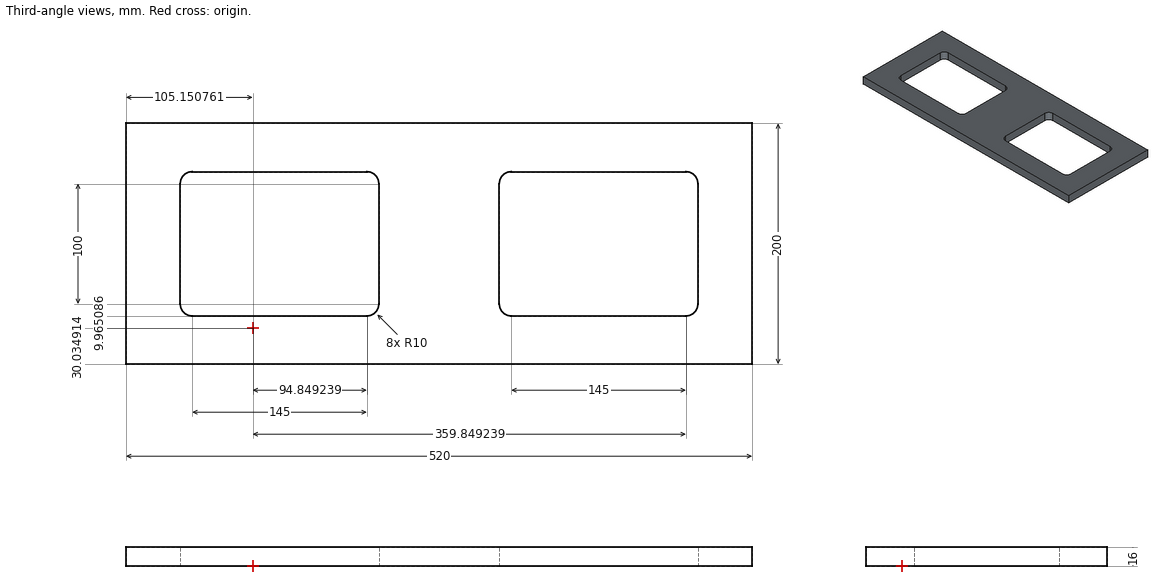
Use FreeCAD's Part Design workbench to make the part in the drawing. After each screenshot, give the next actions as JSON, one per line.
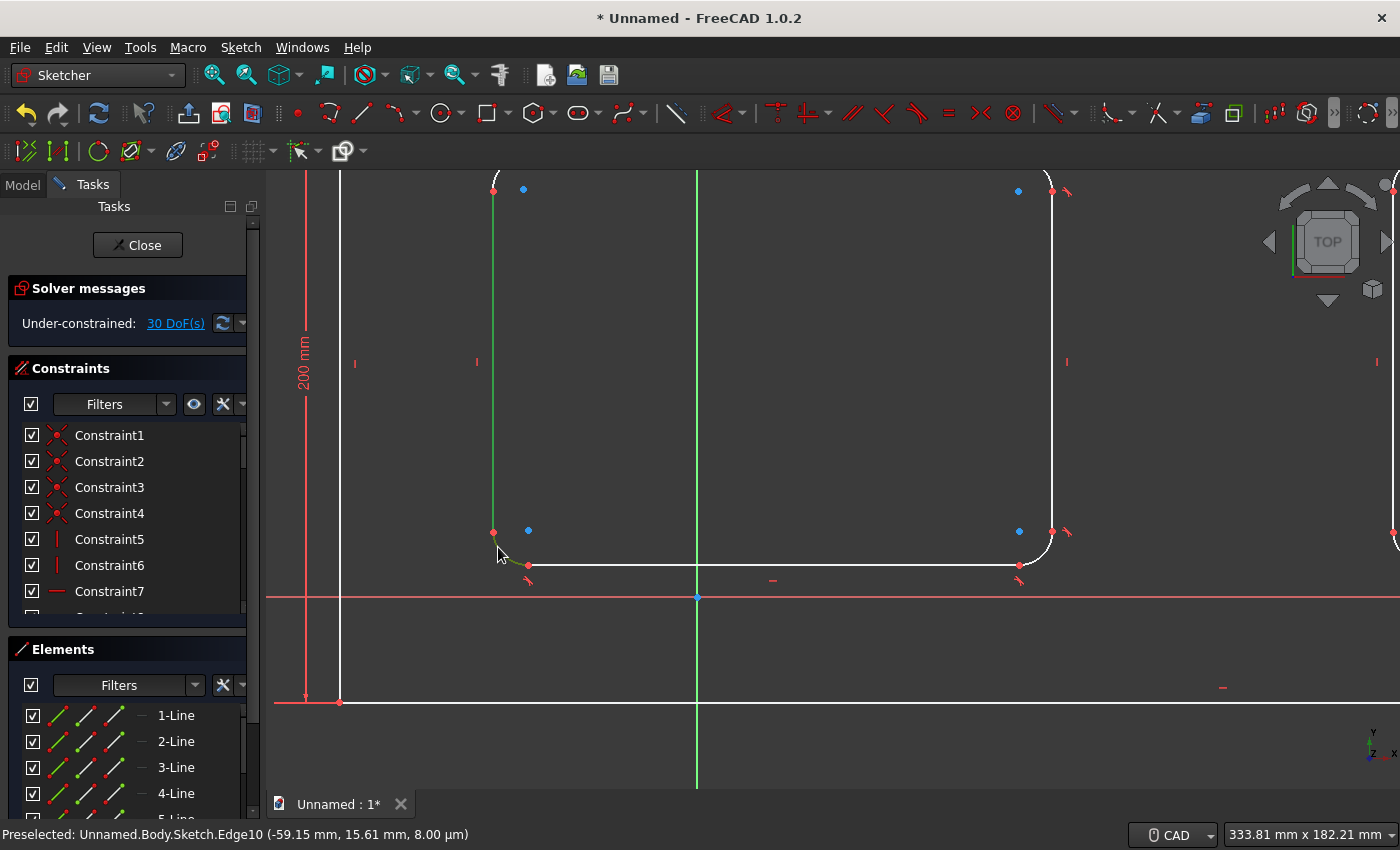
{"action": "key", "text": "t"}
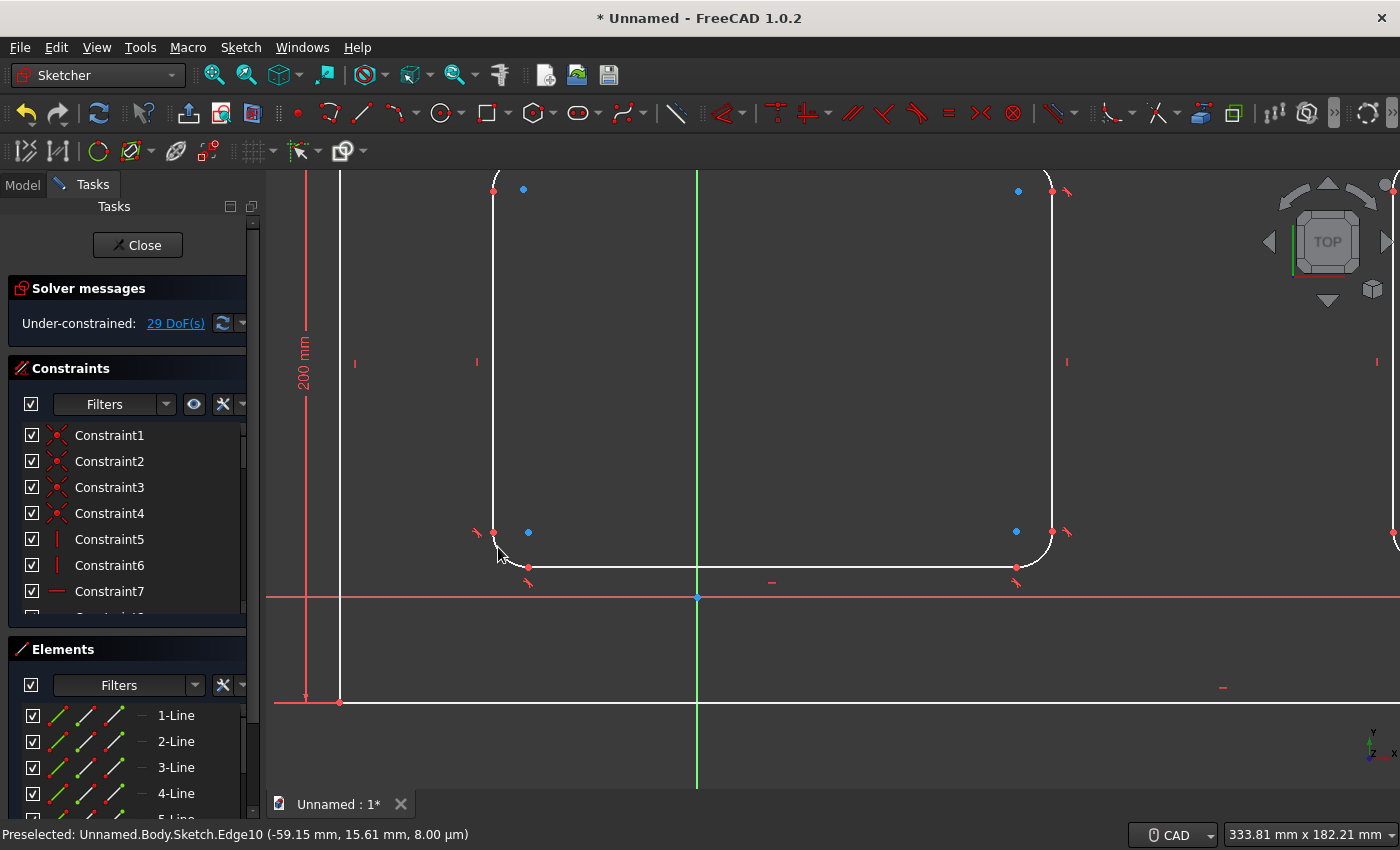
{"action": "left_click", "coordinate": [493, 430]}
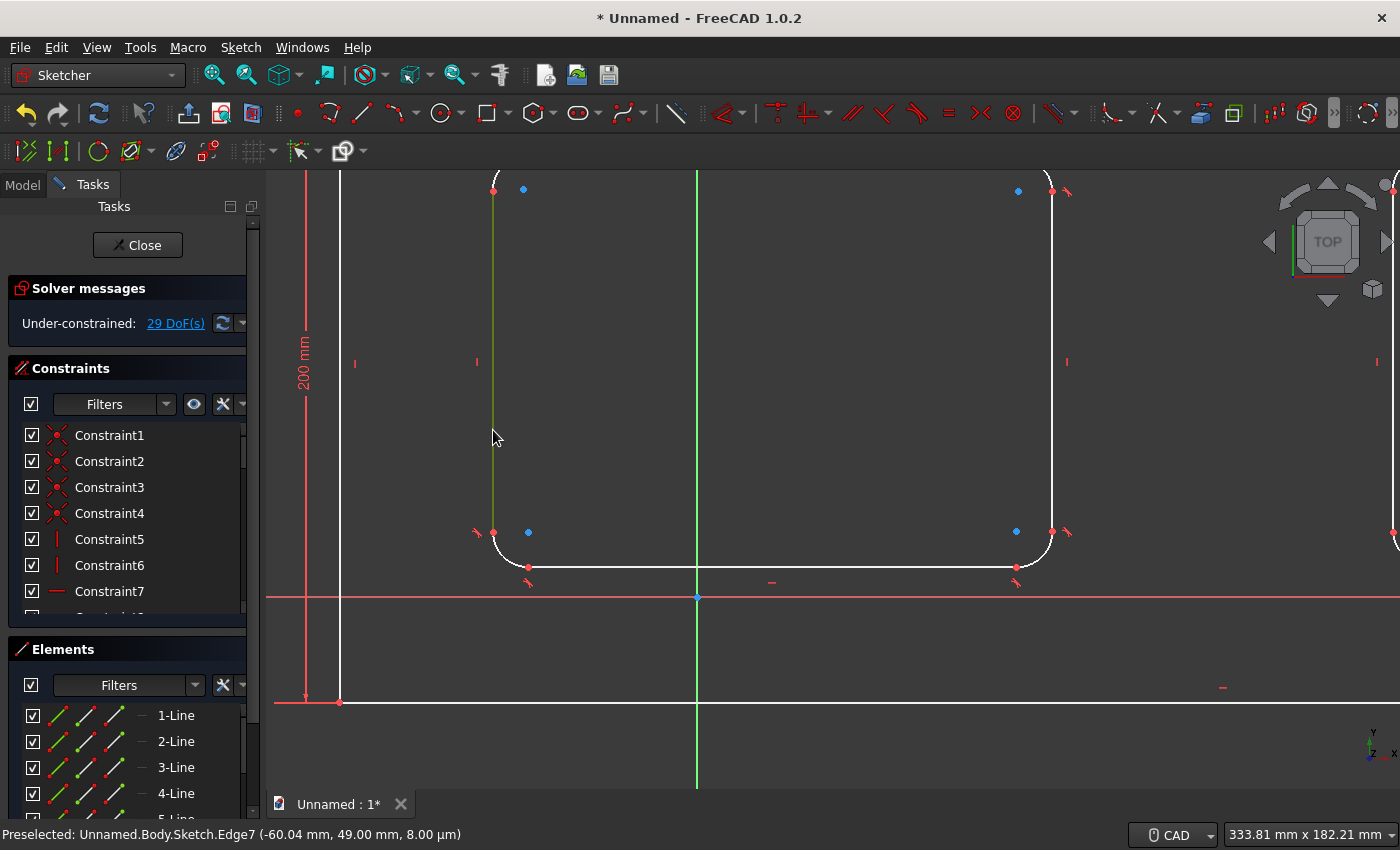
{"action": "scroll", "coordinate": [498, 549], "scroll_direction": "down", "scroll_amount": 5}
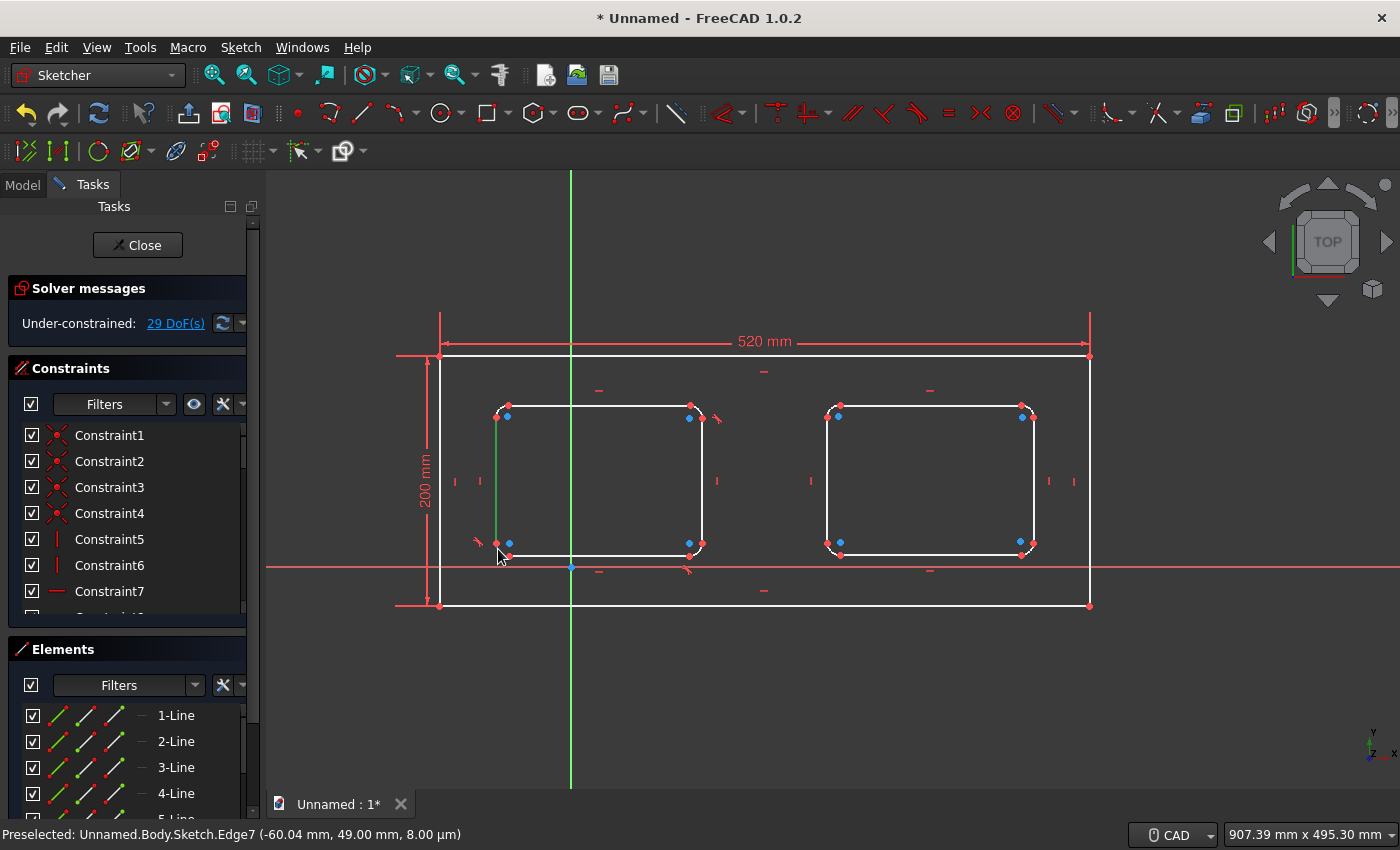
{"action": "scroll", "coordinate": [503, 407], "scroll_direction": "up", "scroll_amount": 5}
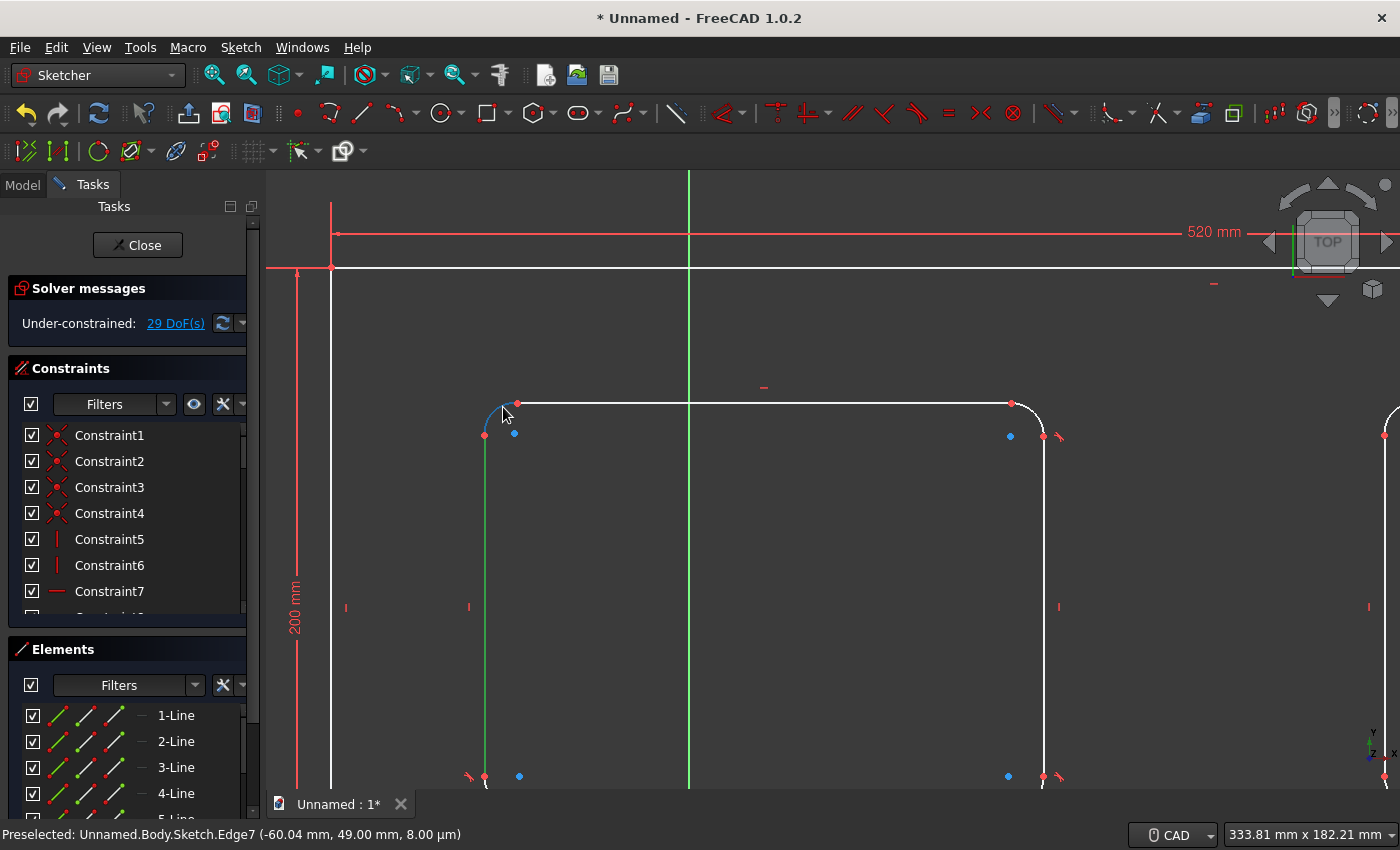
{"action": "left_click", "coordinate": [502, 406]}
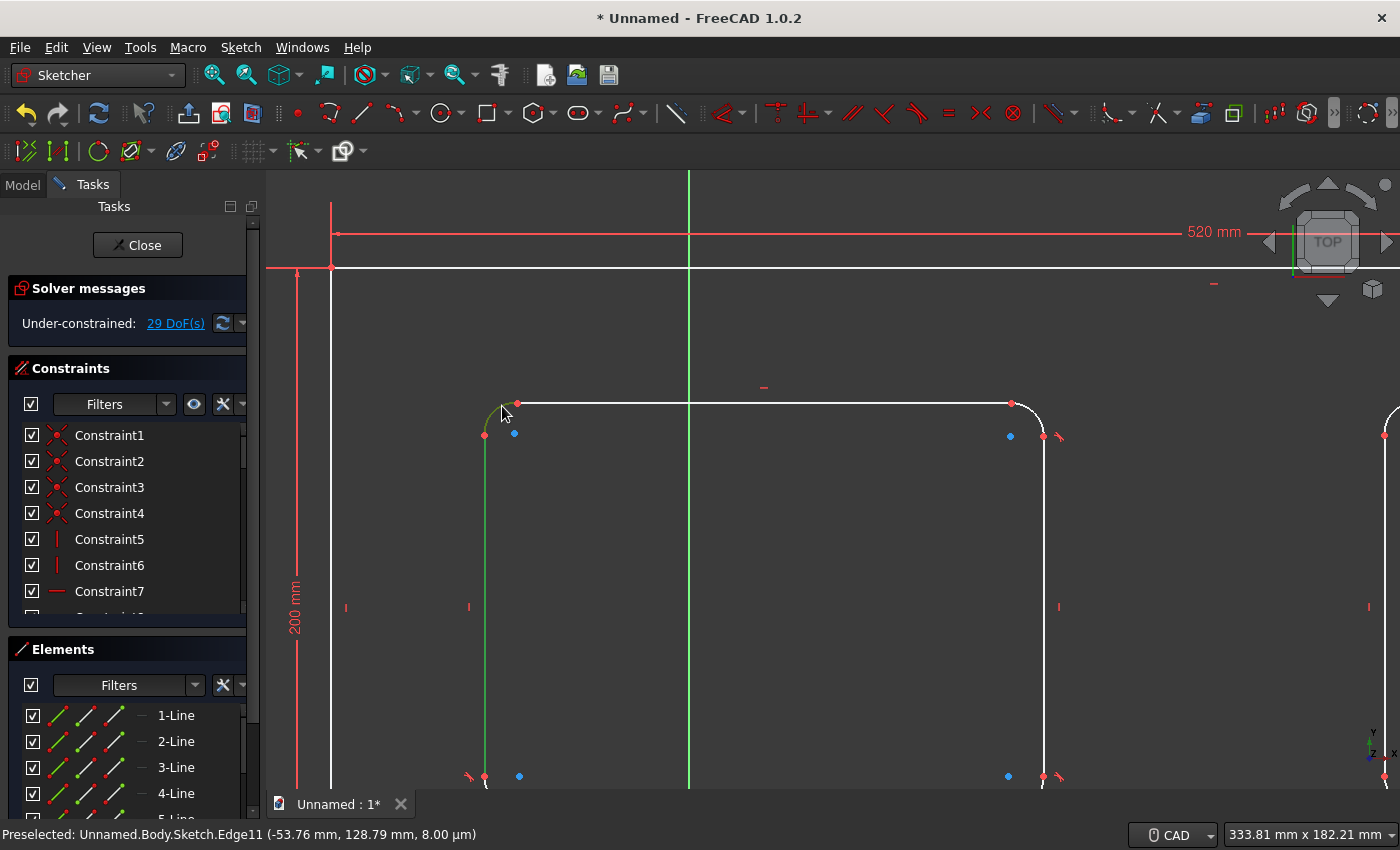
{"action": "key", "text": "t"}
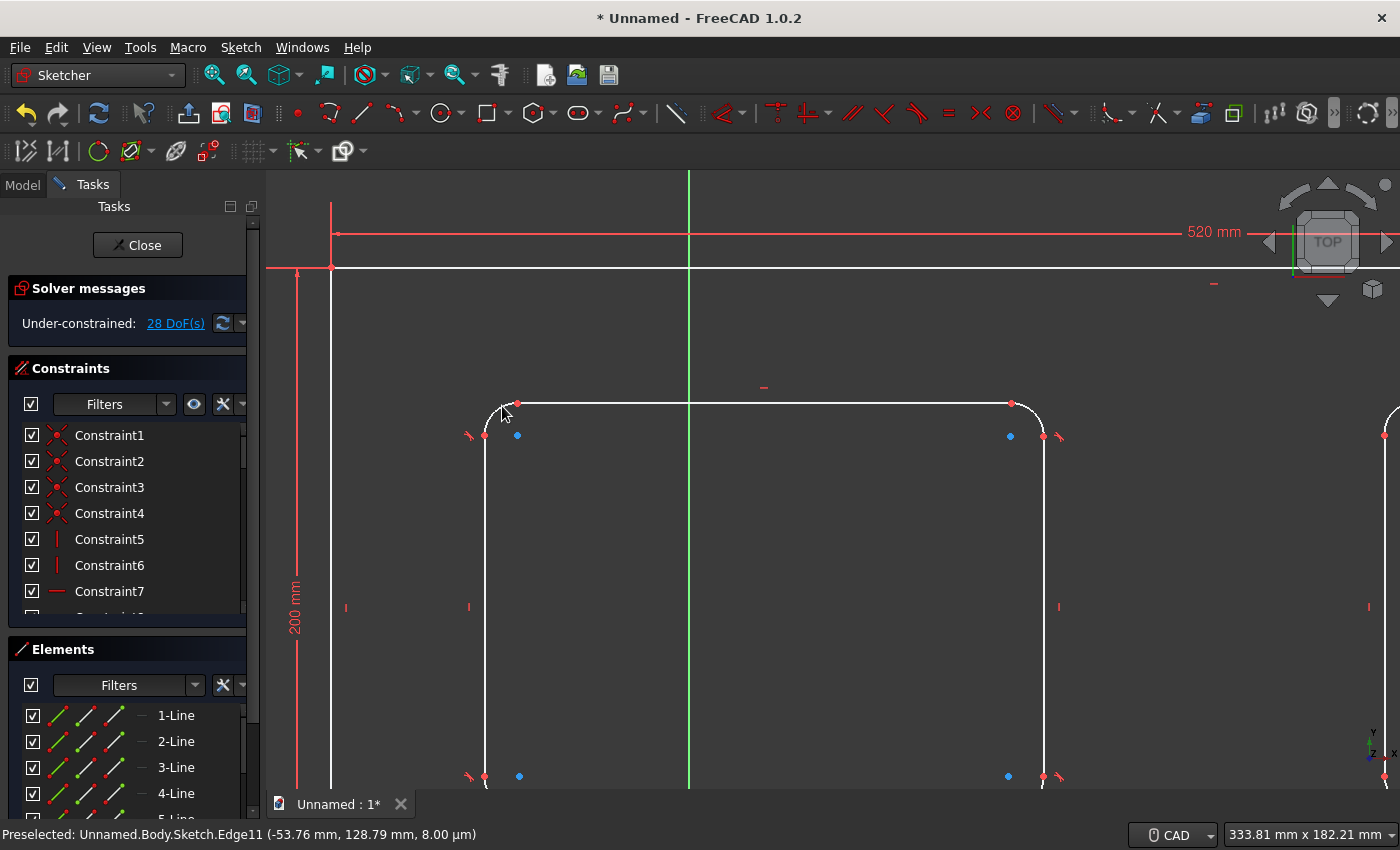
{"action": "left_click", "coordinate": [666, 403]}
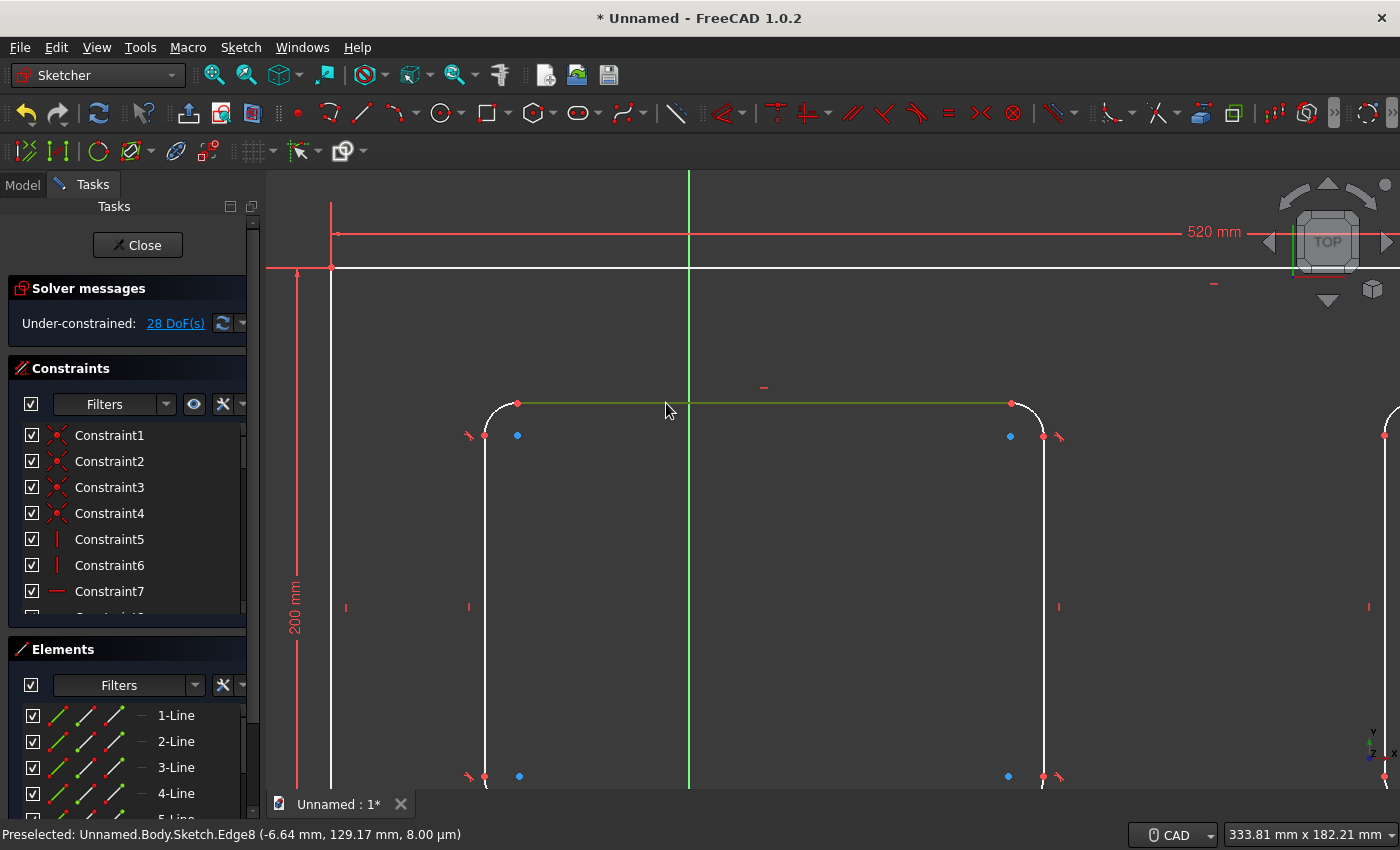
{"action": "left_click", "coordinate": [502, 407]}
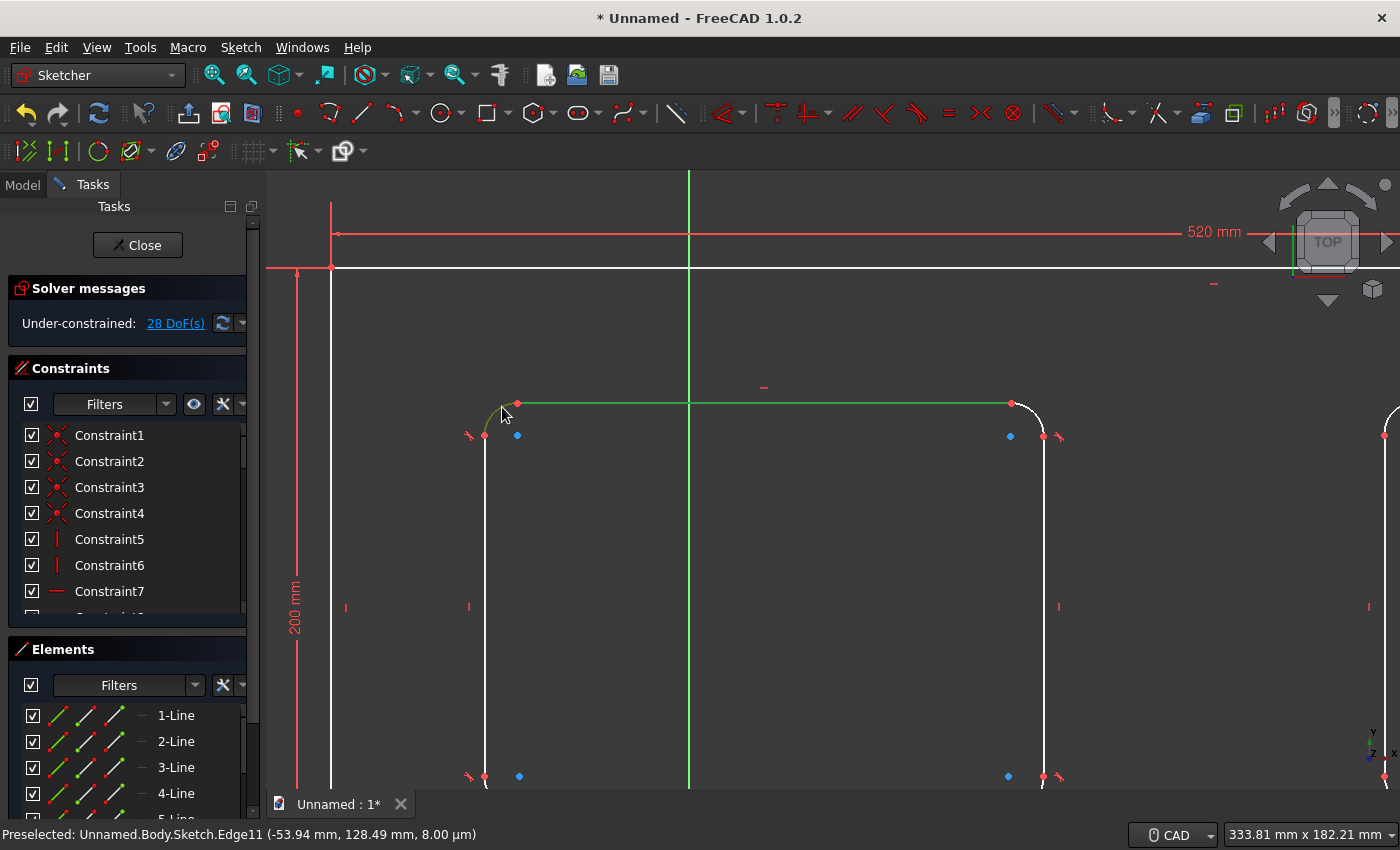
{"action": "key", "text": "t"}